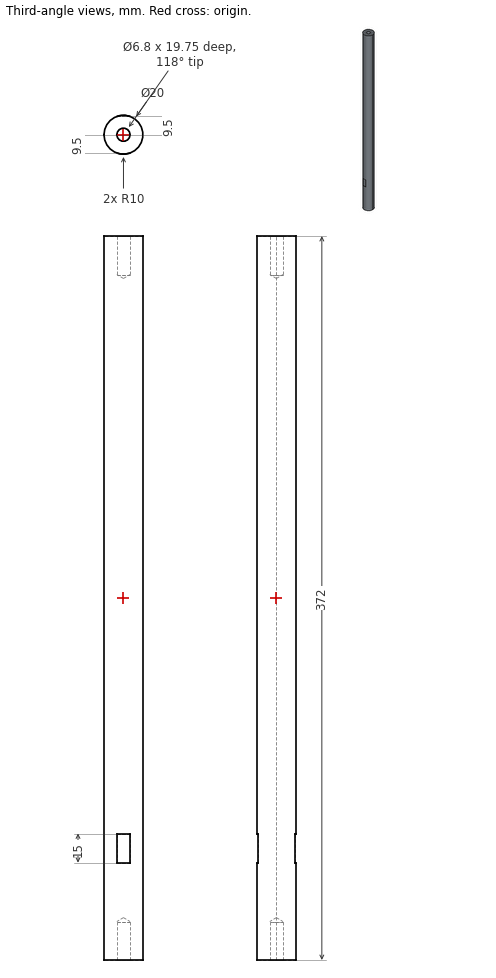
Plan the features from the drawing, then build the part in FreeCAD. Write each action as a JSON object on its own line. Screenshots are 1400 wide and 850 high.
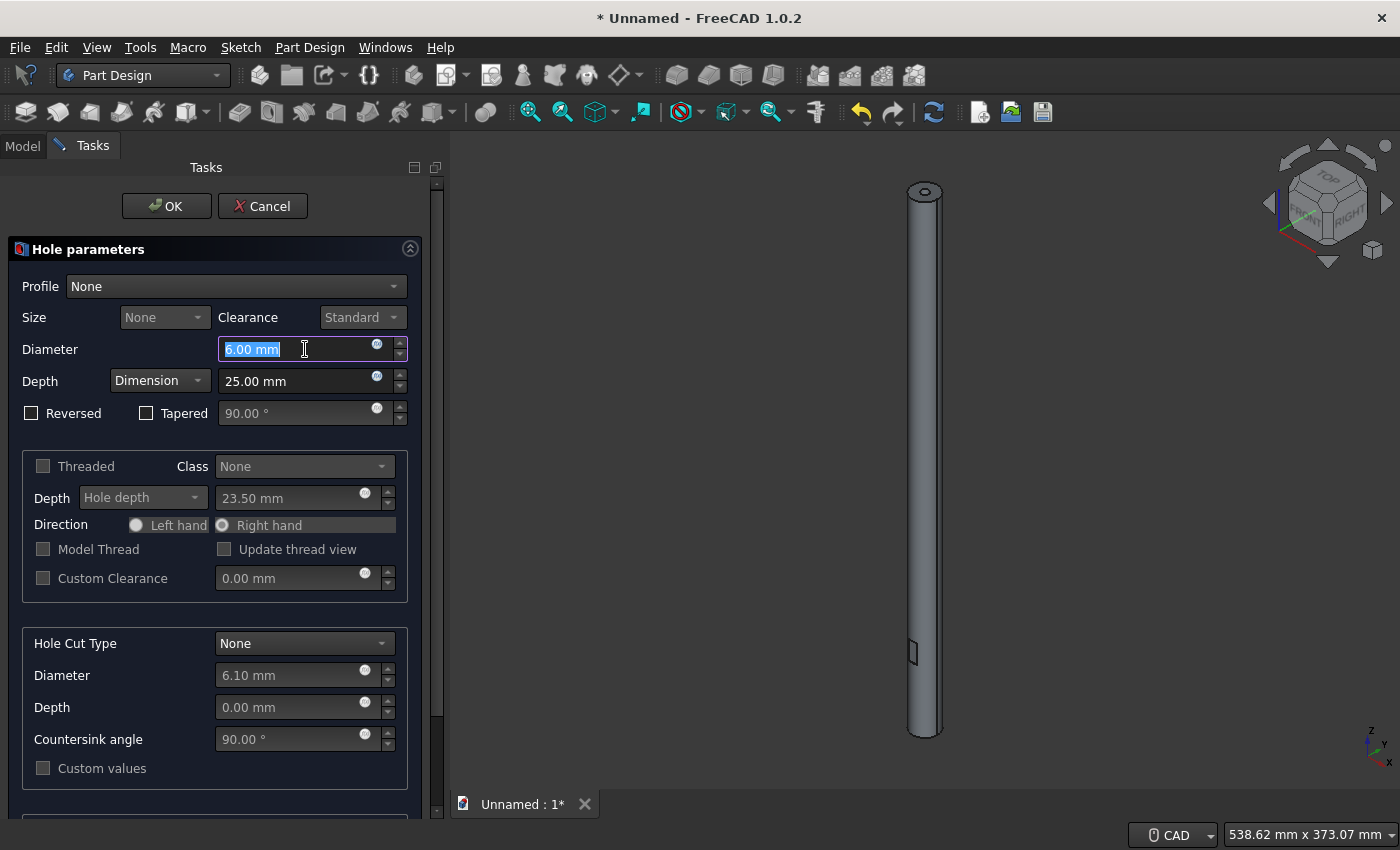
{"action": "type", "text": "6.8"}
{"action": "key", "text": "Tab"}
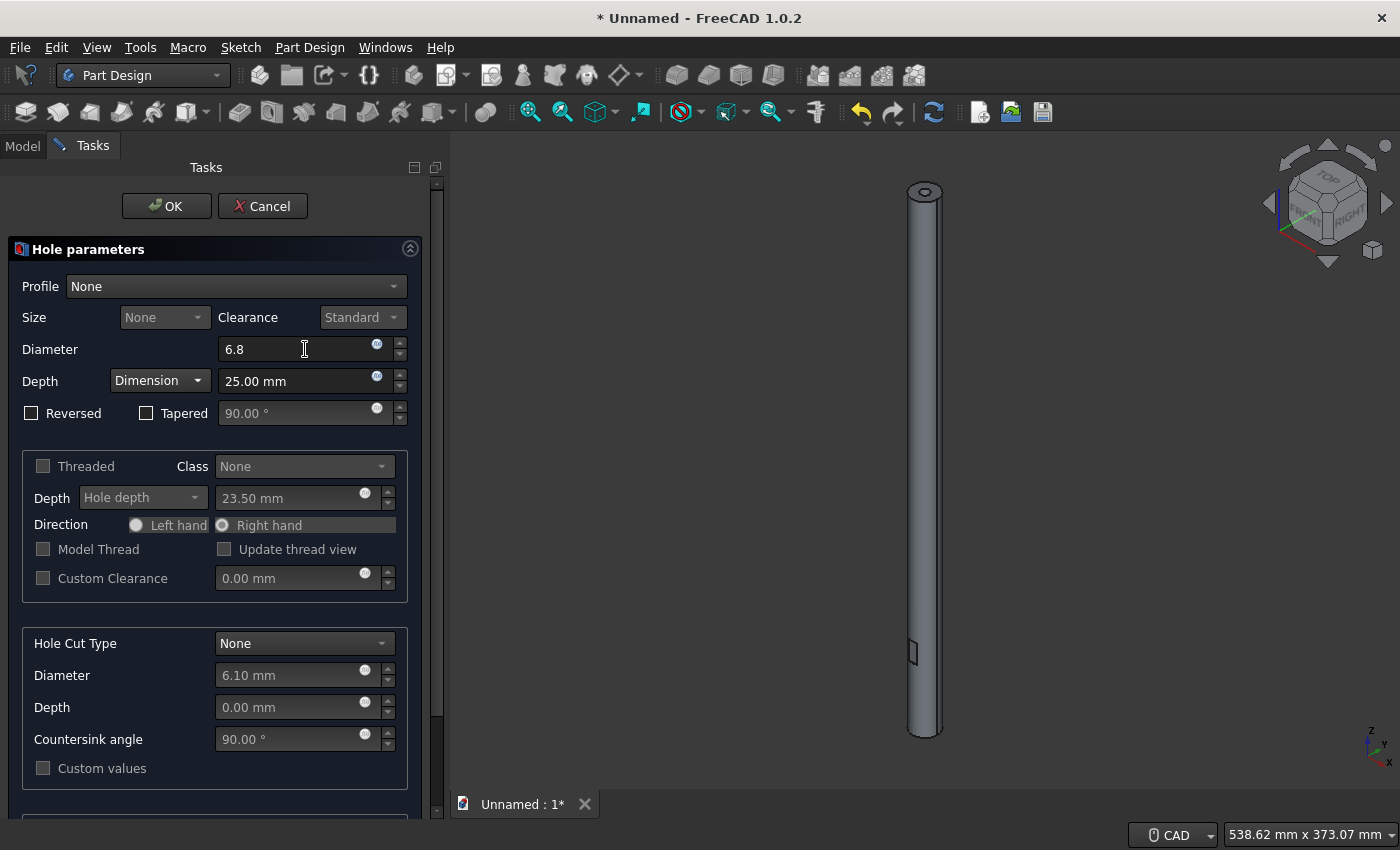
{"action": "triple_click", "coordinate": [305, 381]}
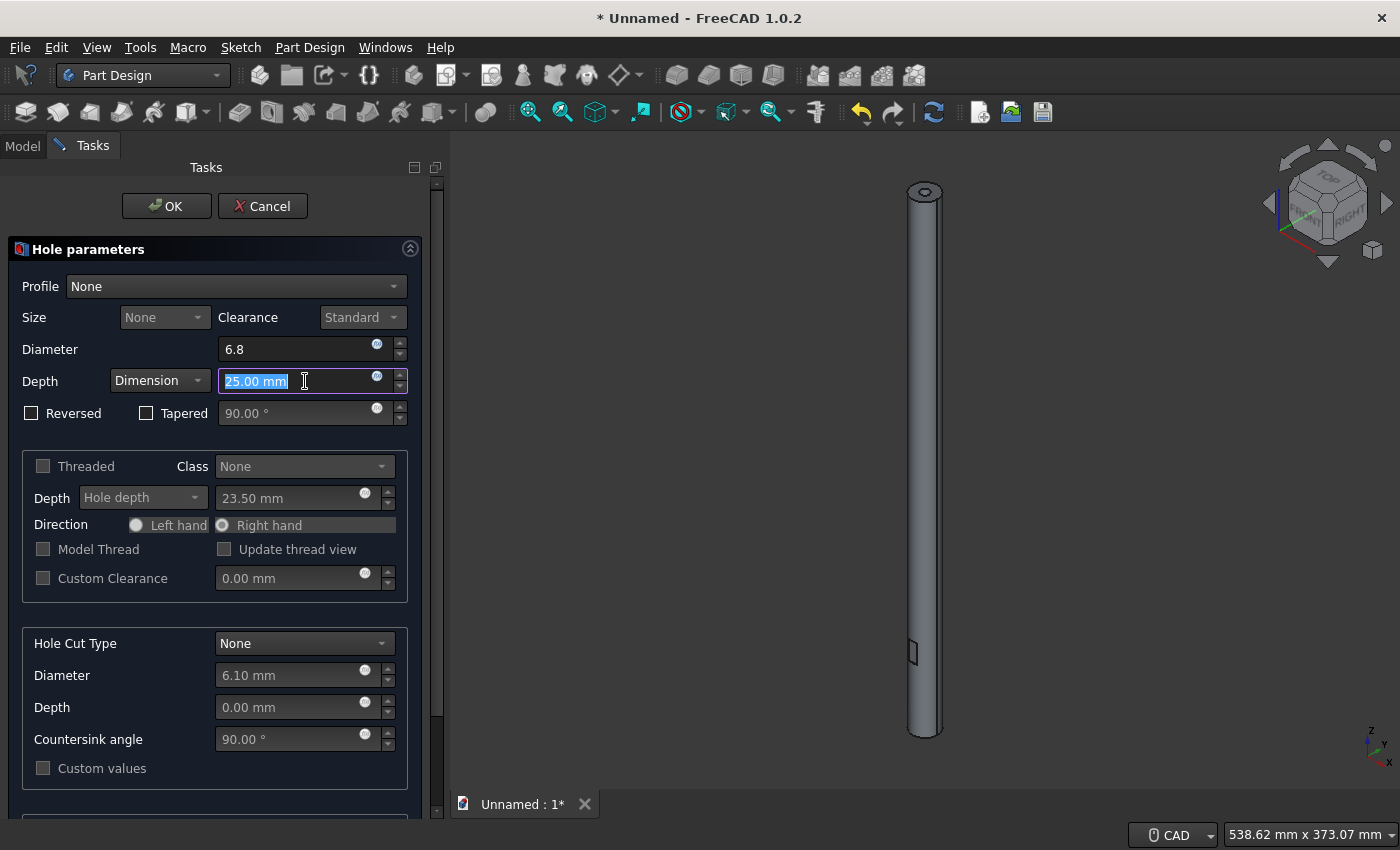
{"action": "type", "text": "19.75"}
{"action": "key", "text": "Tab"}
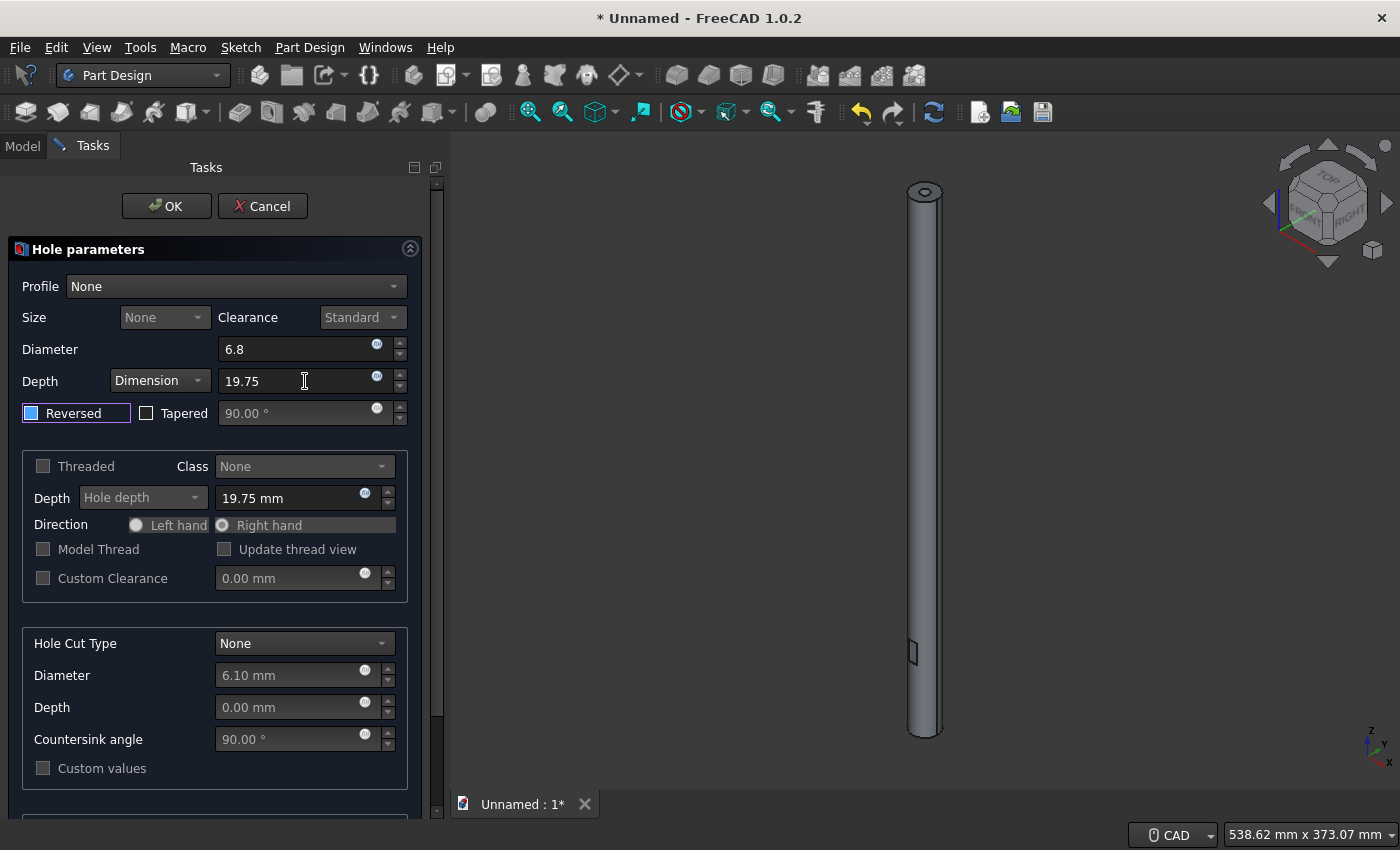
{"action": "left_click", "coordinate": [167, 206]}